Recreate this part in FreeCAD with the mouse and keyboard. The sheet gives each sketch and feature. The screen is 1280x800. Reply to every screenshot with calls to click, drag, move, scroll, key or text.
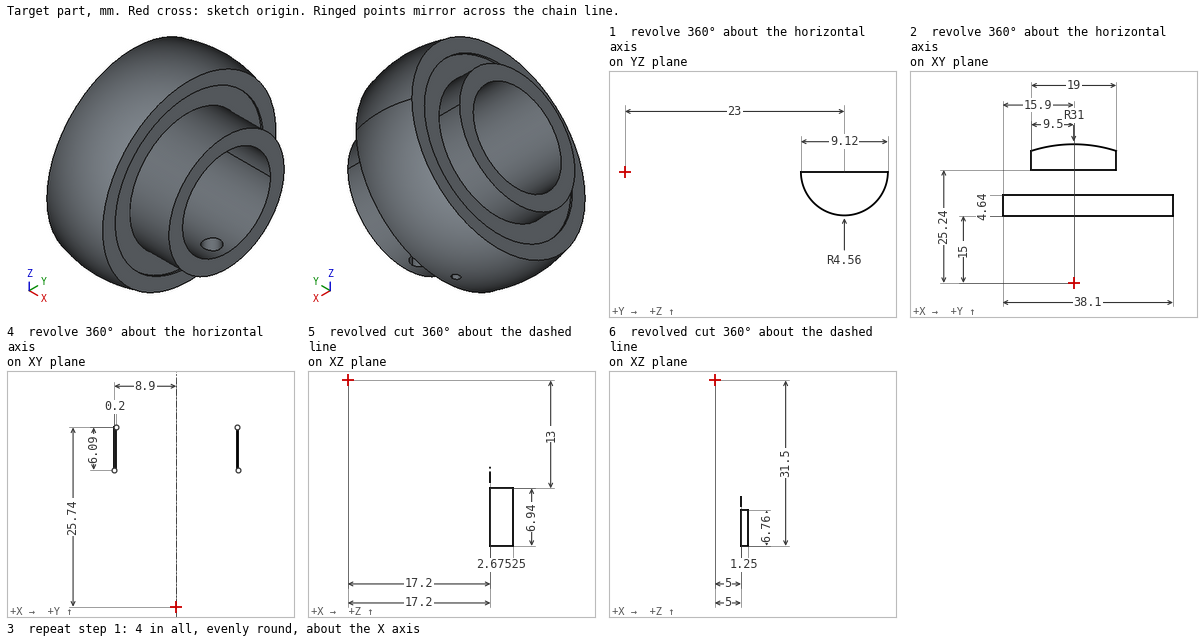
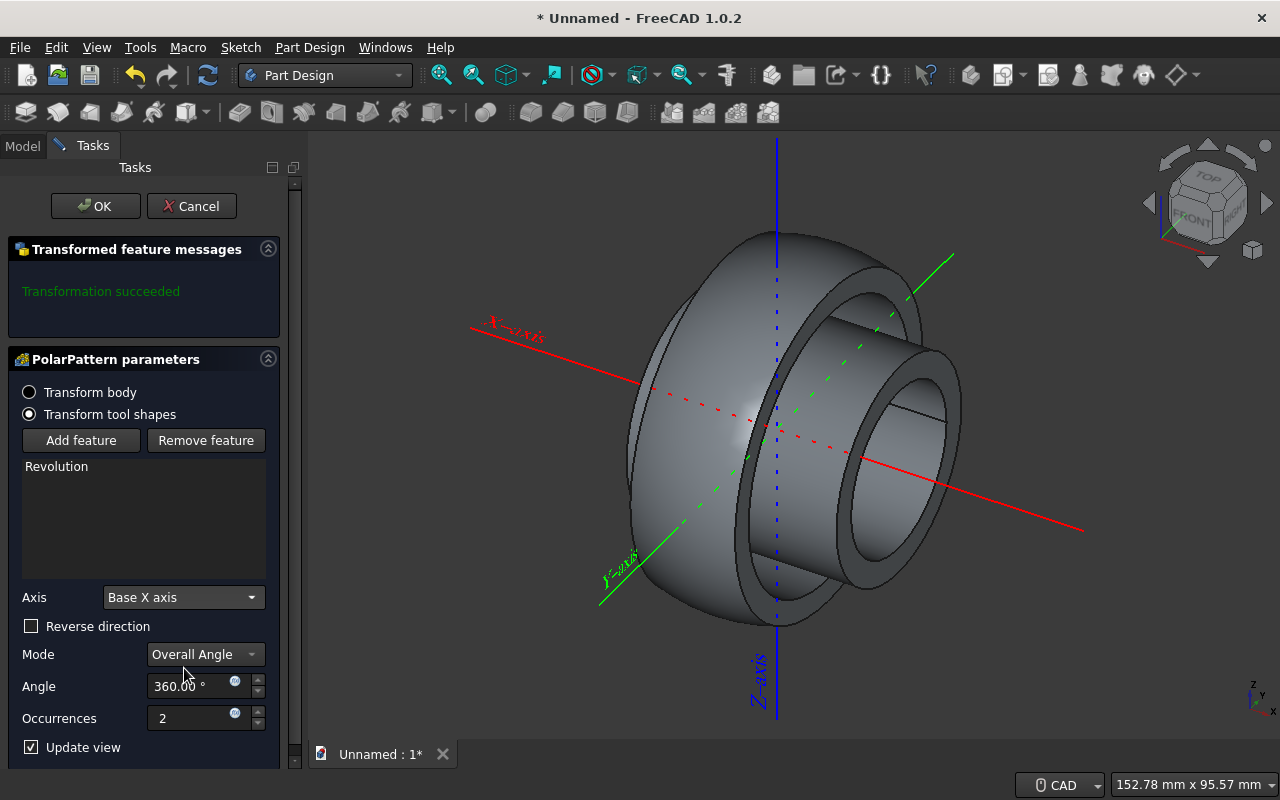
triple_click(198, 718)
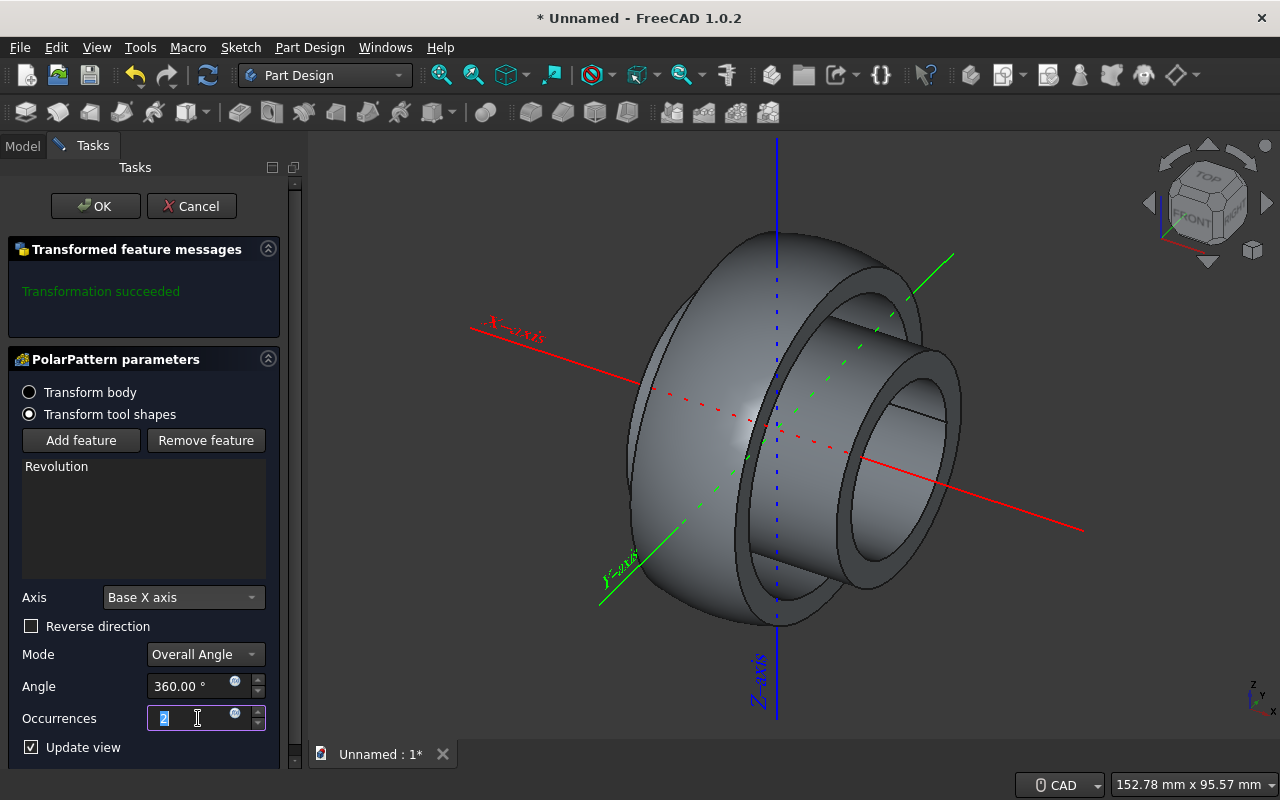
text(4)
key(Tab)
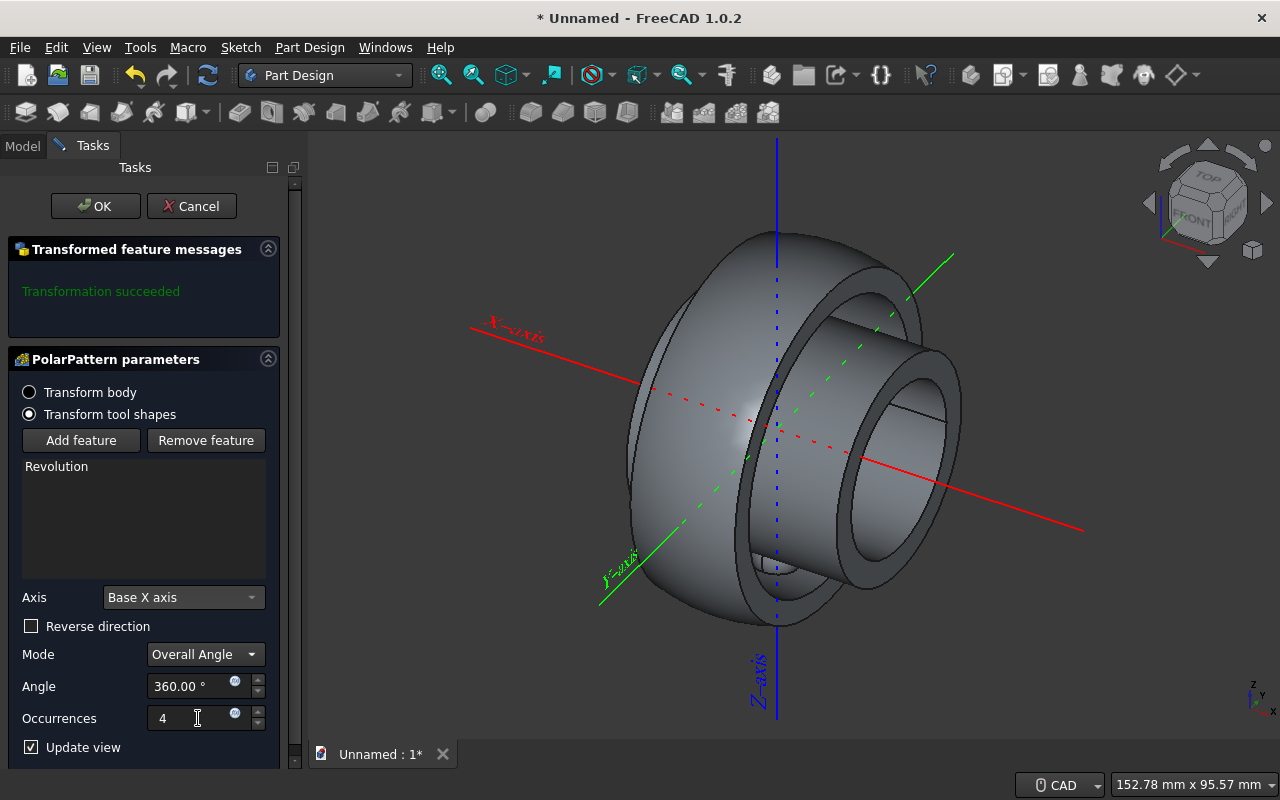
click(96, 206)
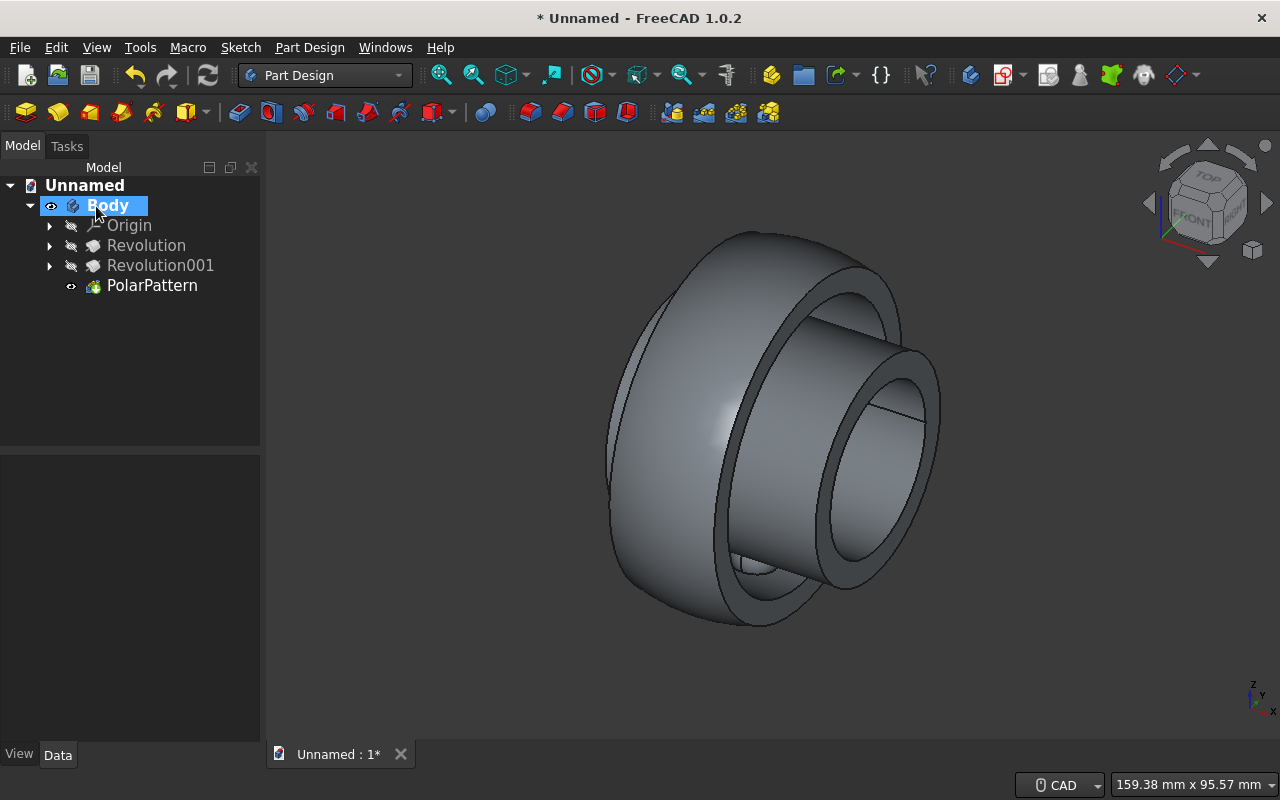
click(1004, 76)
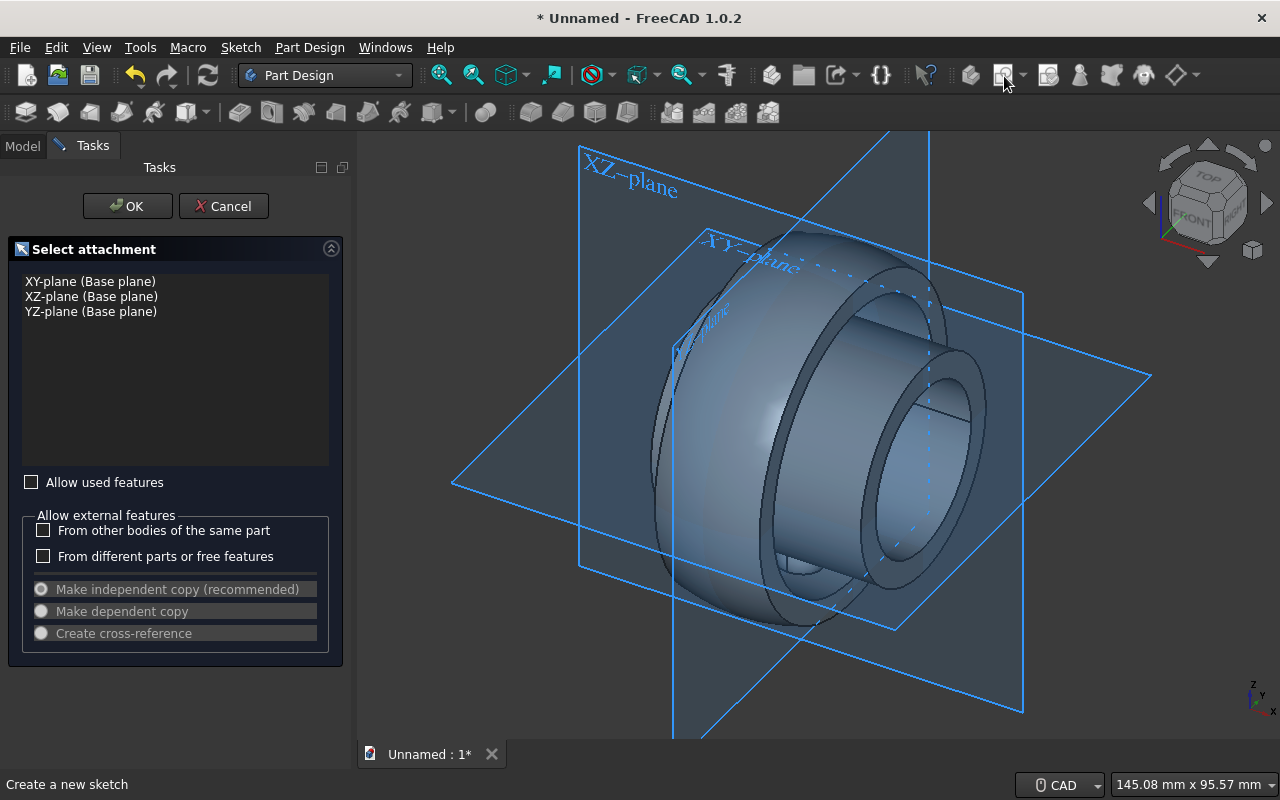
click(82, 282)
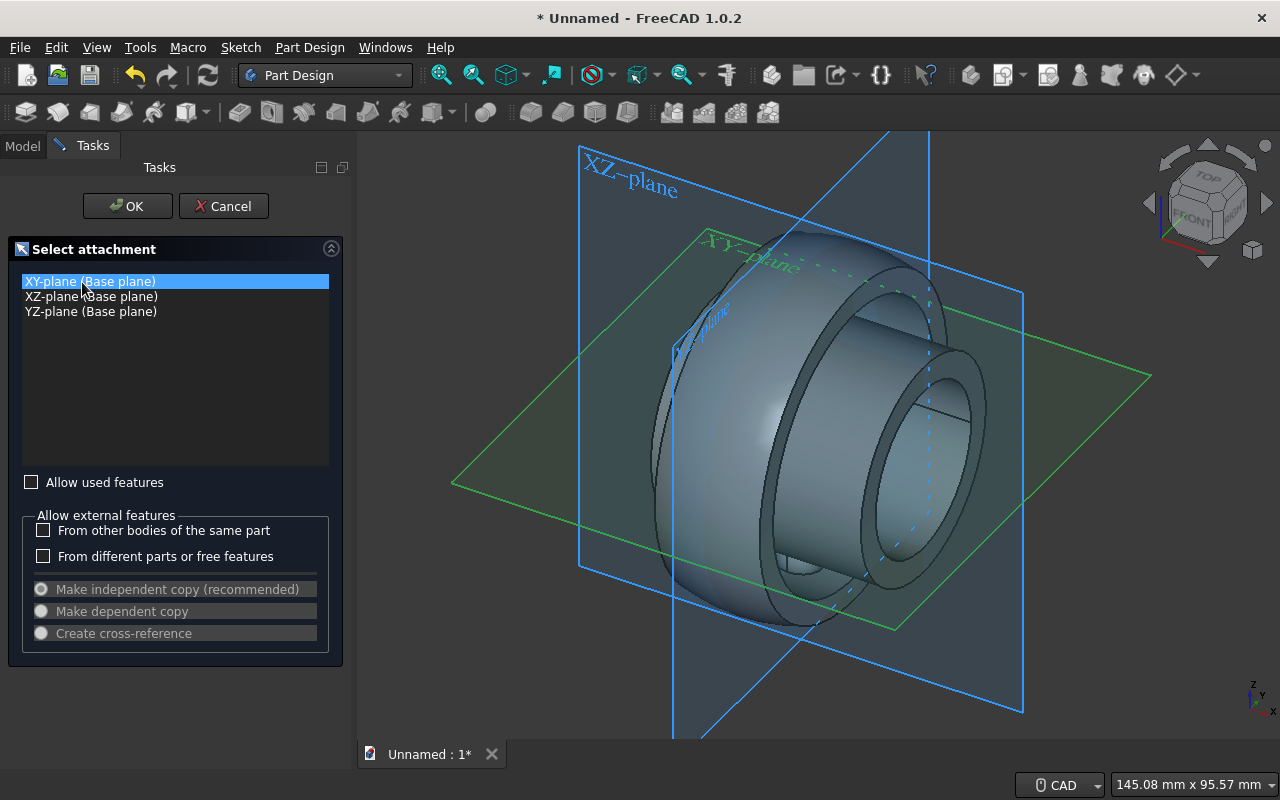
click(128, 206)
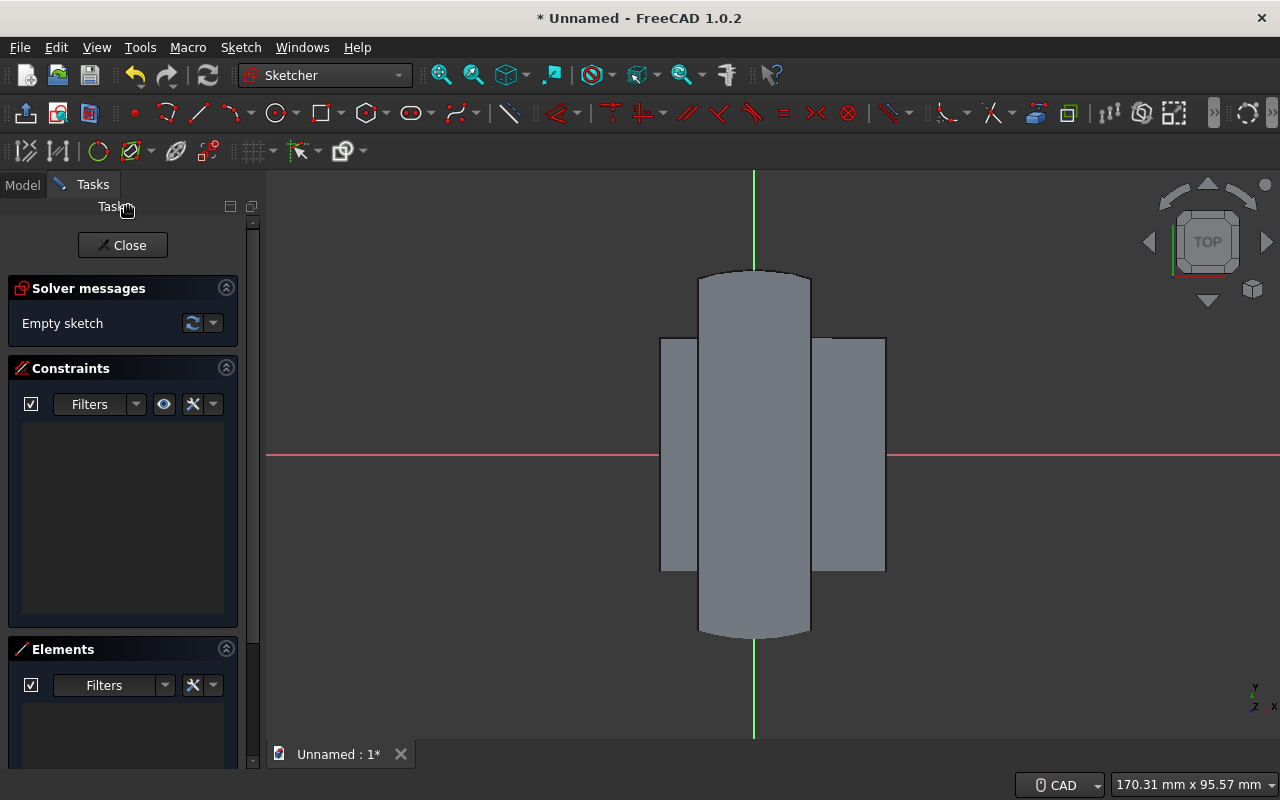
click(90, 114)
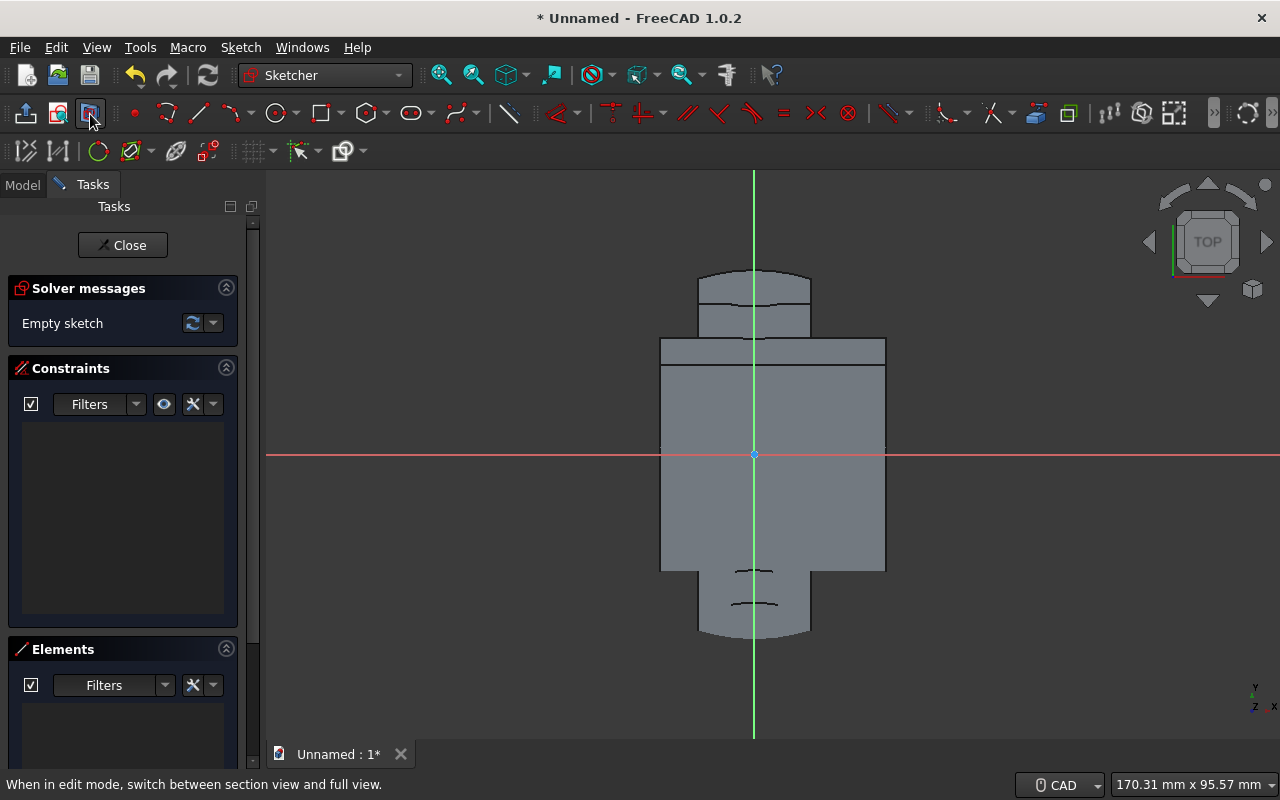
scroll(795, 316, up, 4)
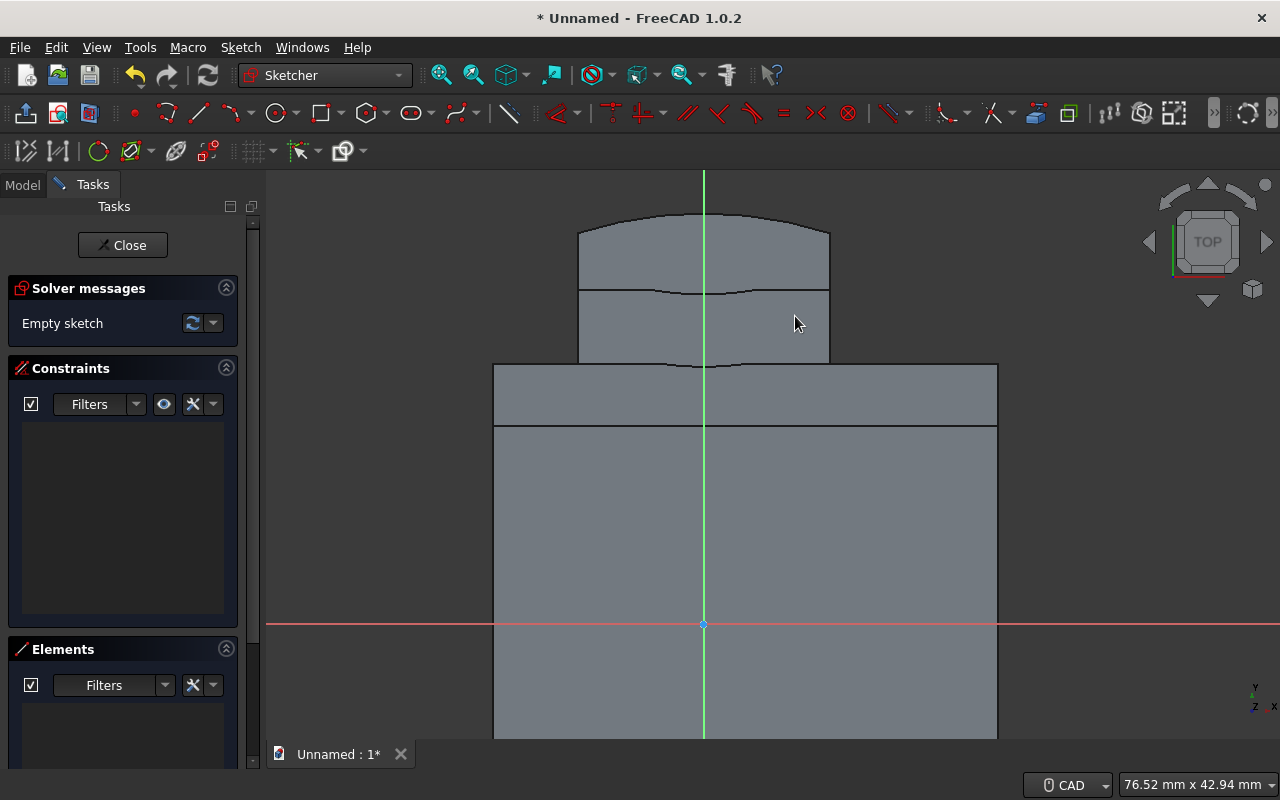
click(322, 114)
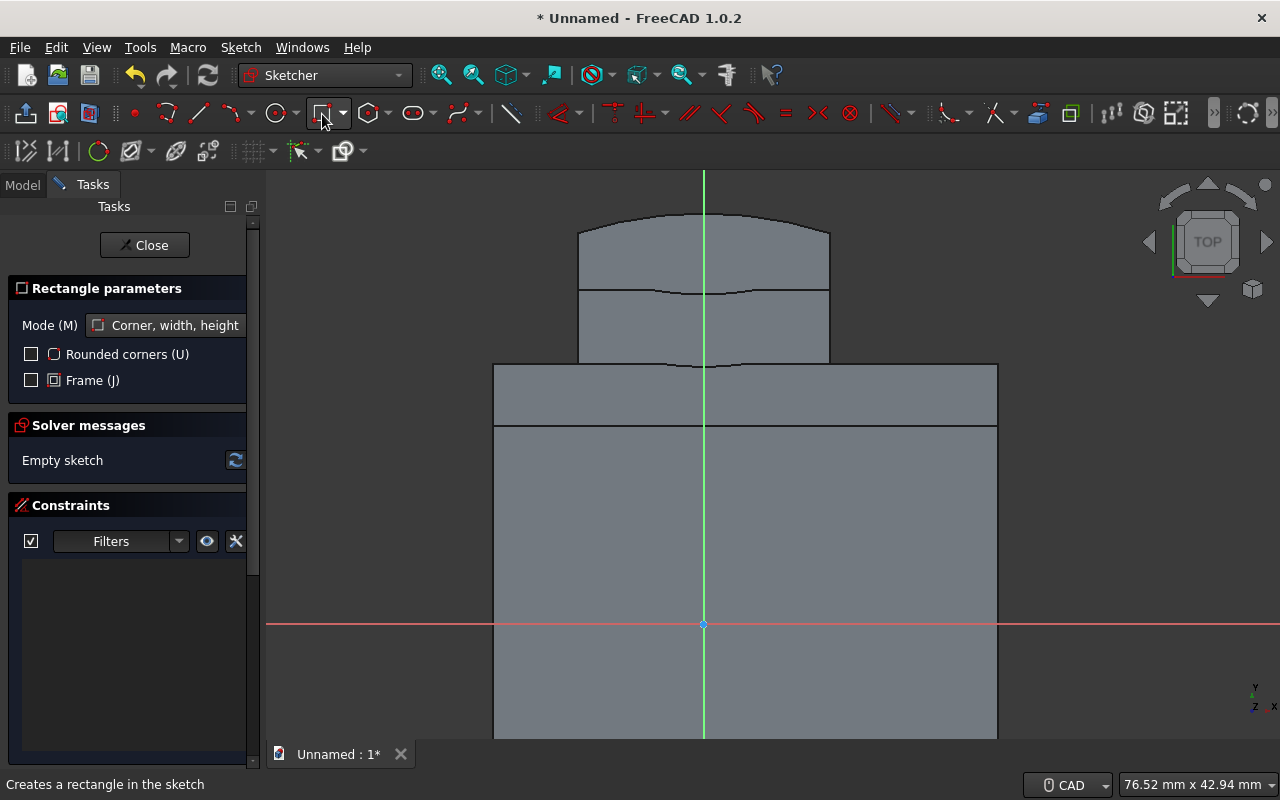
scroll(586, 283, up, 9)